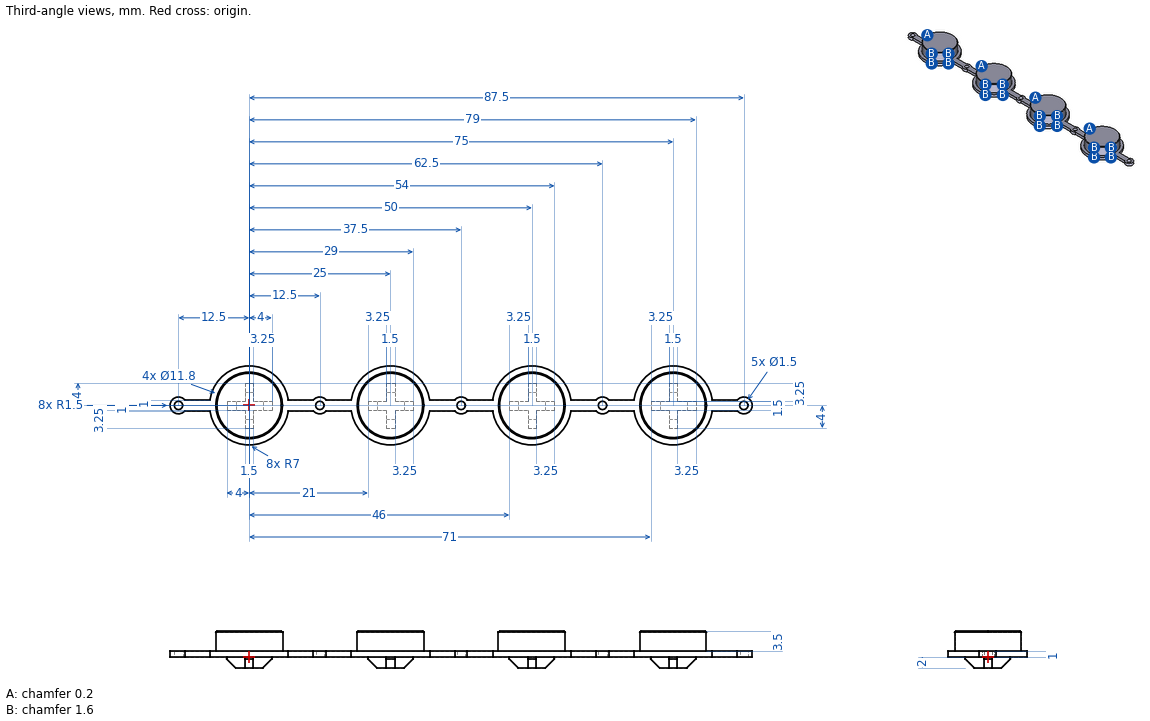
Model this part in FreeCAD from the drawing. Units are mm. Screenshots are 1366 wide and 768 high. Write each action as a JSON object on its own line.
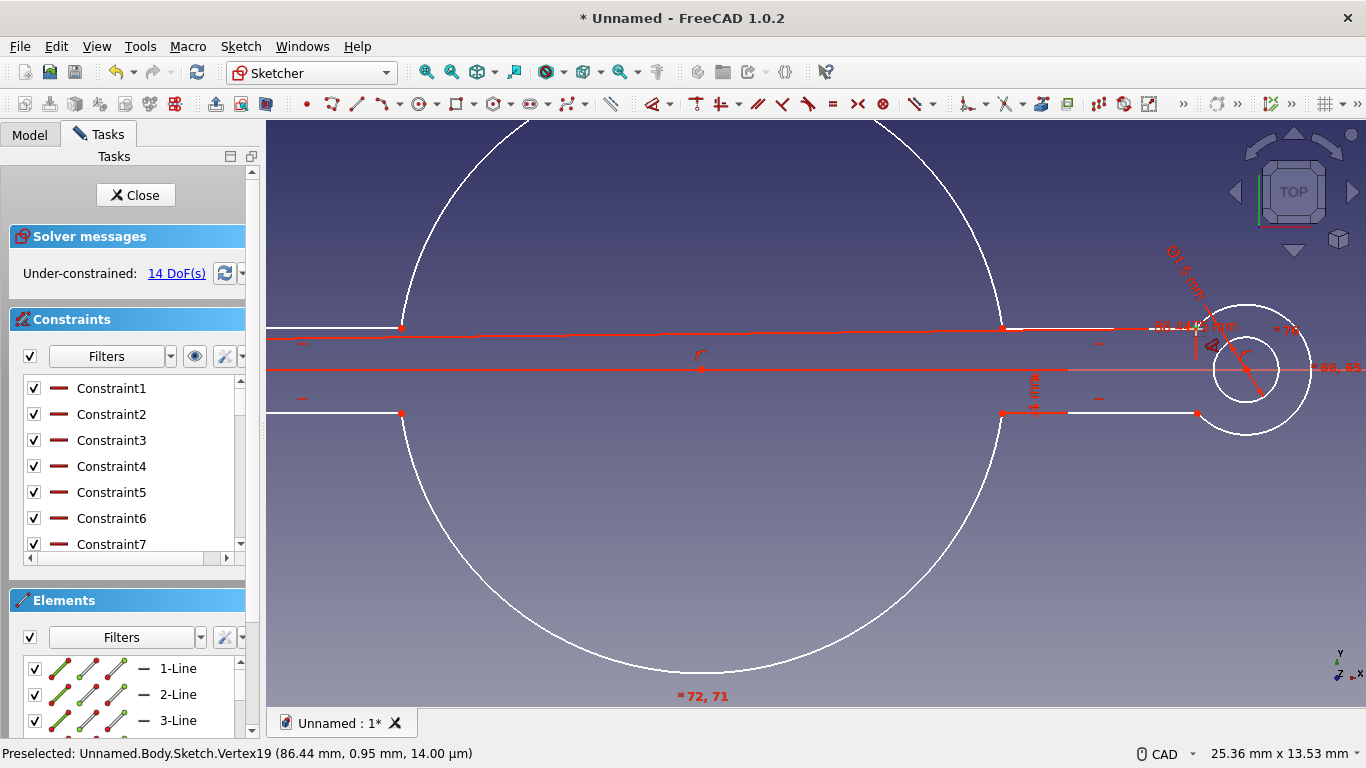
{"action": "key", "text": "Escape"}
{"action": "key", "text": "Escape"}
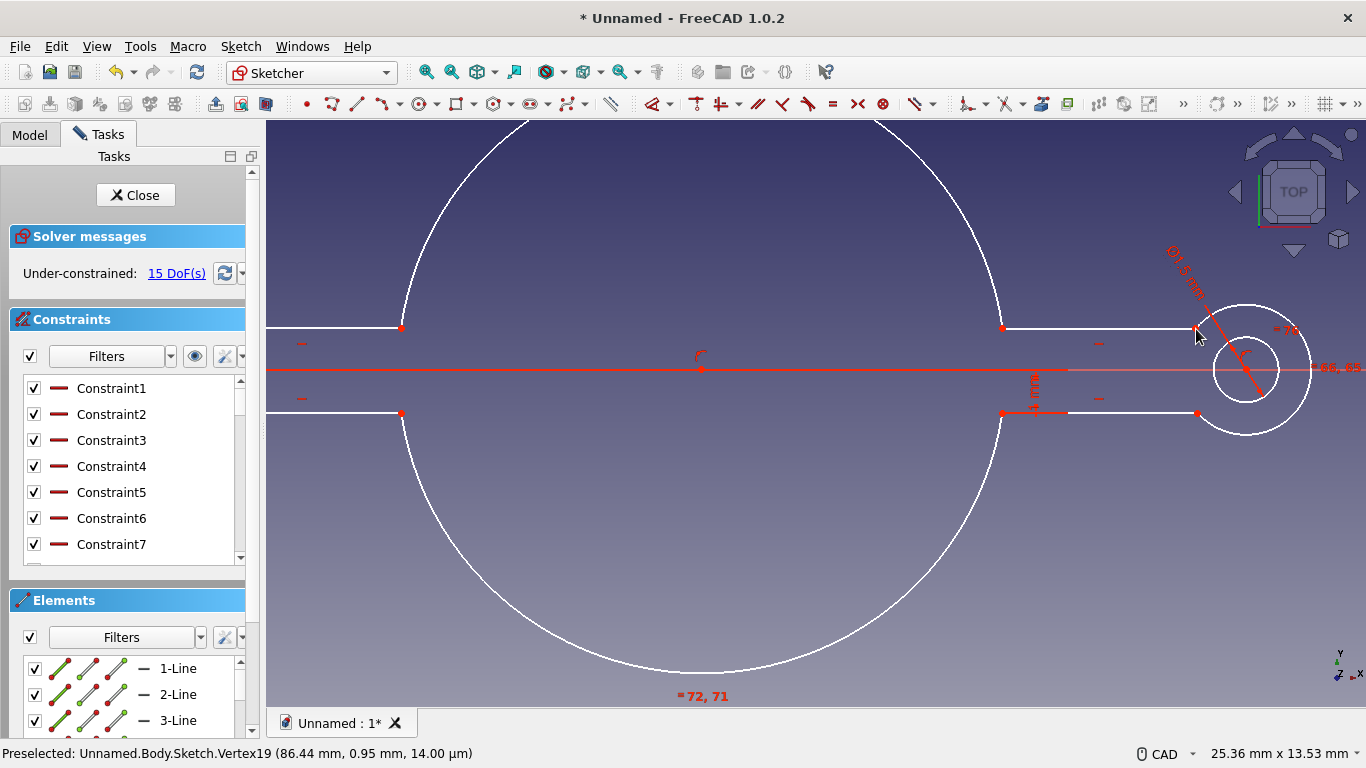
{"action": "left_click", "coordinate": [1196, 329]}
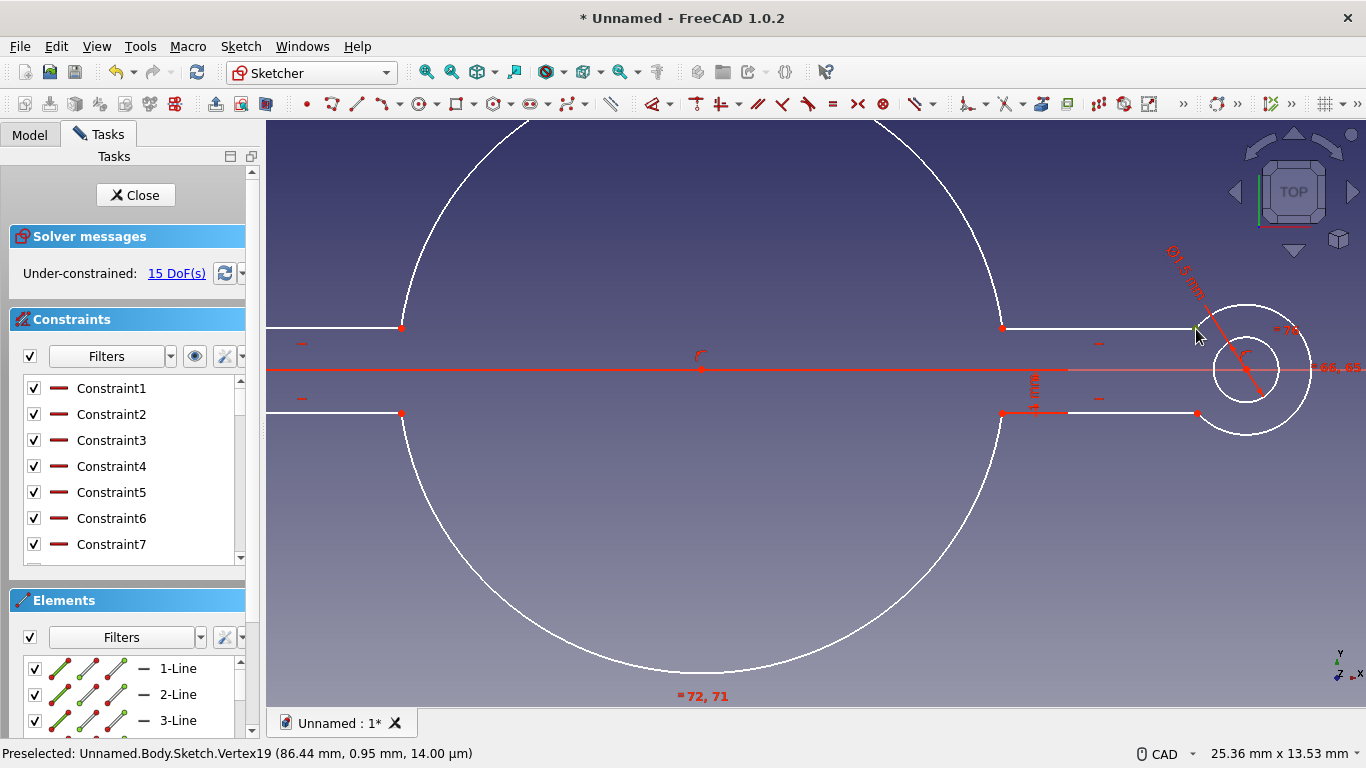
{"action": "key", "text": "i"}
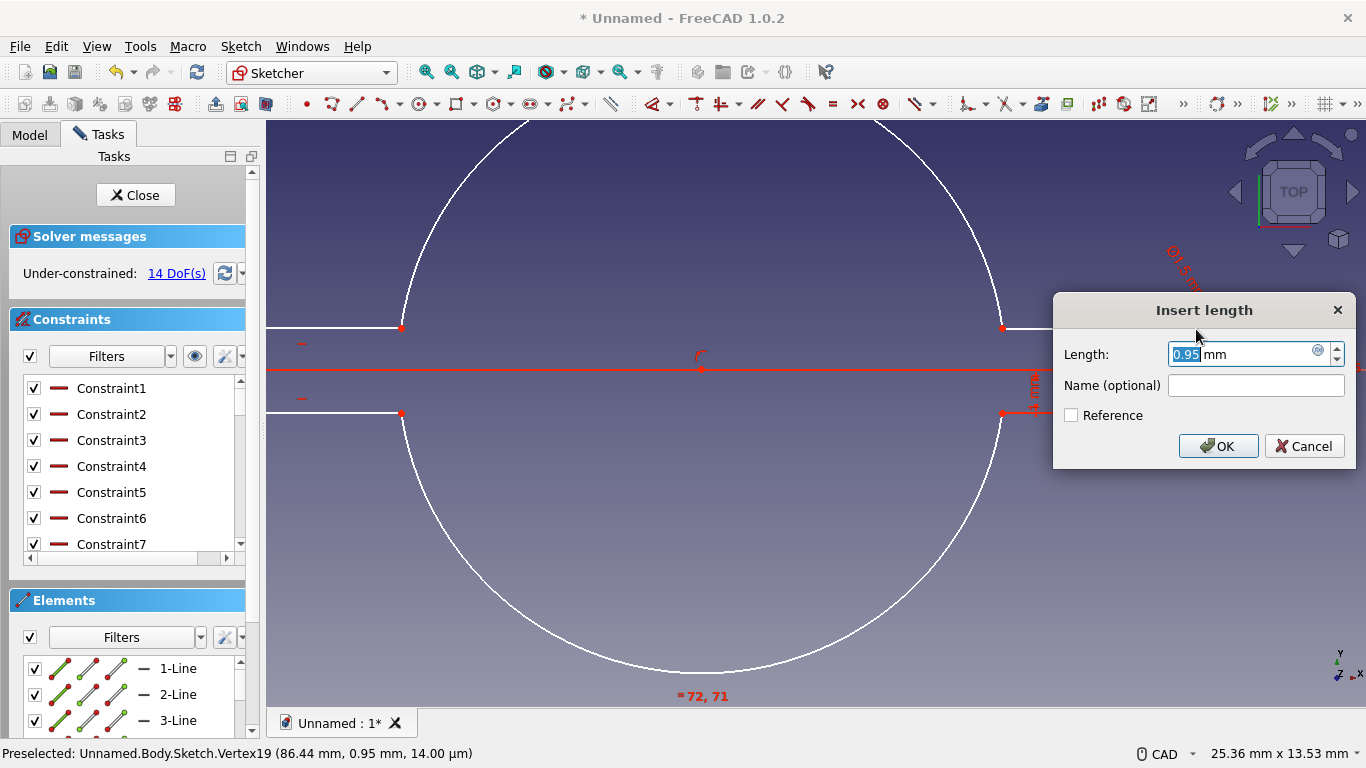
{"action": "type", "text": "1"}
{"action": "key", "text": "Return"}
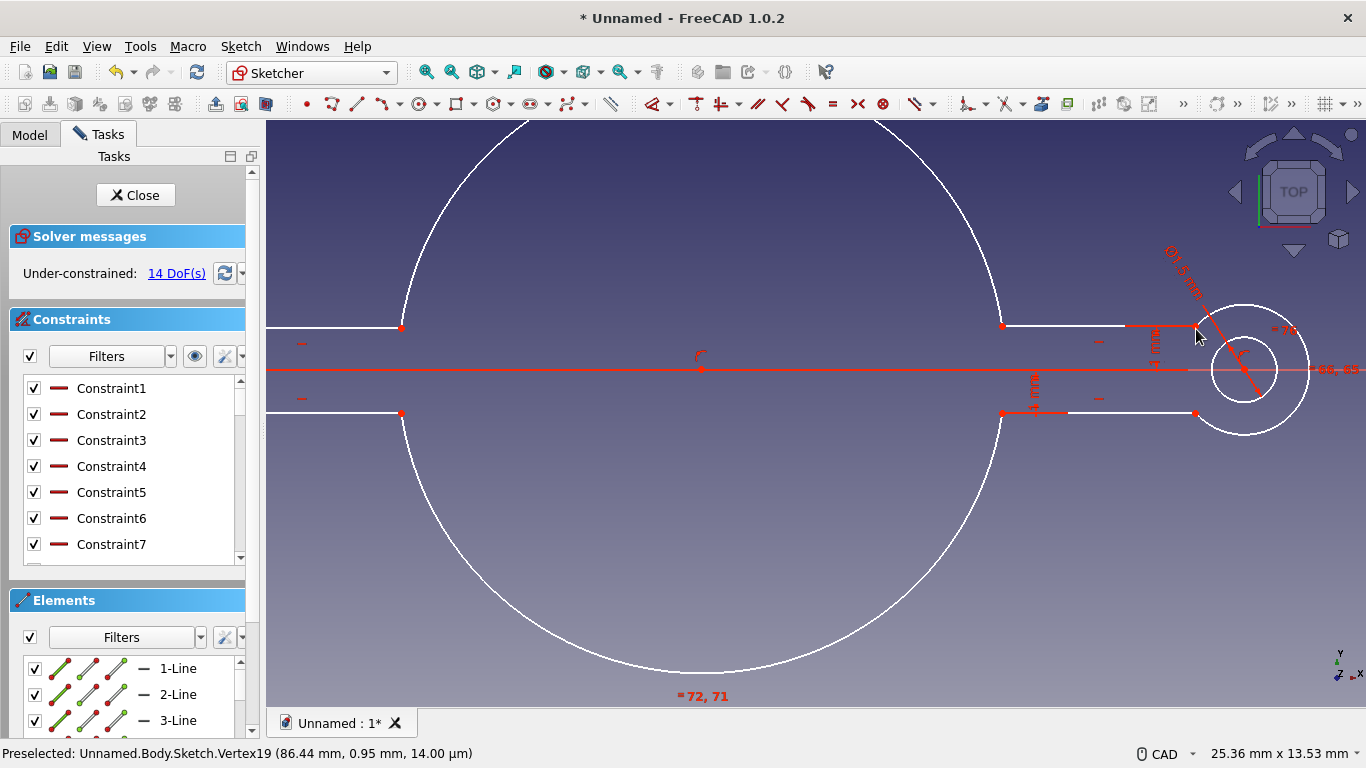
{"action": "left_click", "coordinate": [401, 328]}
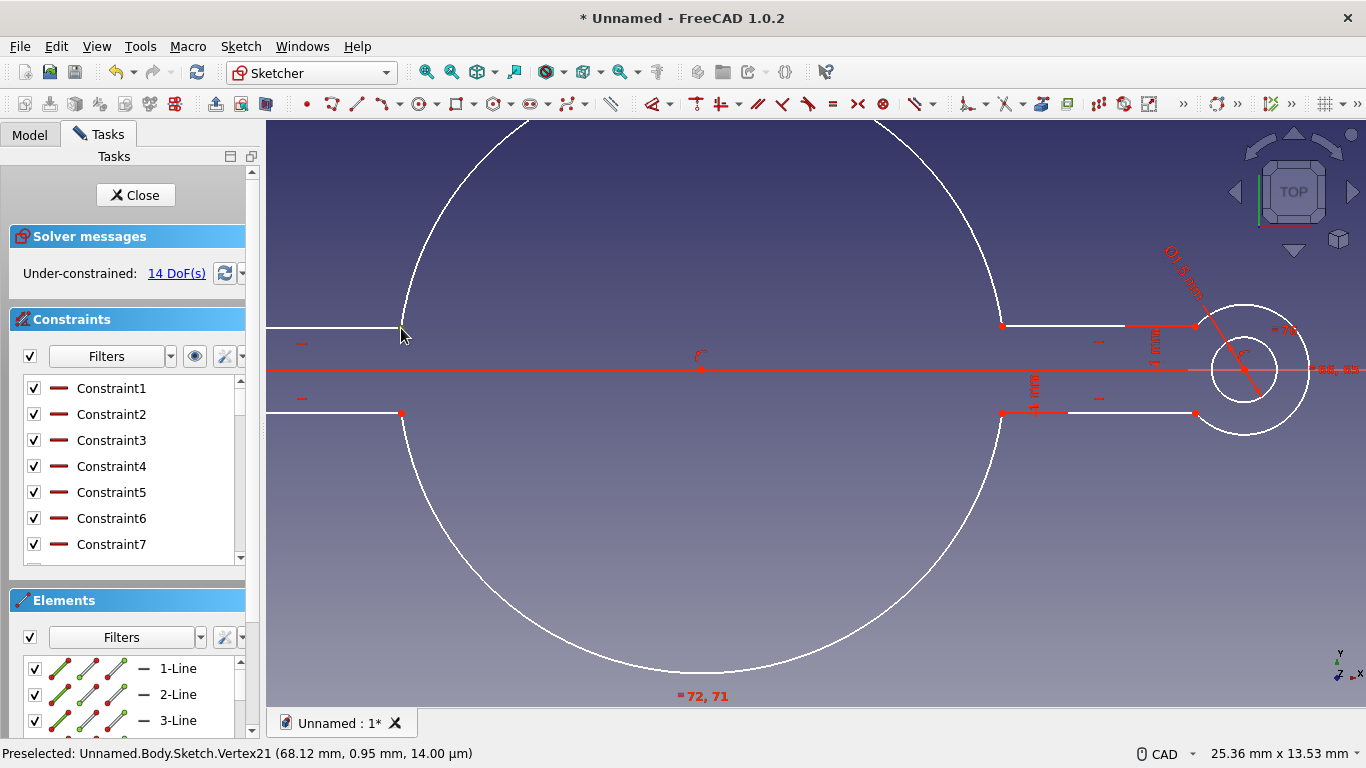
{"action": "left_click", "coordinate": [670, 104]}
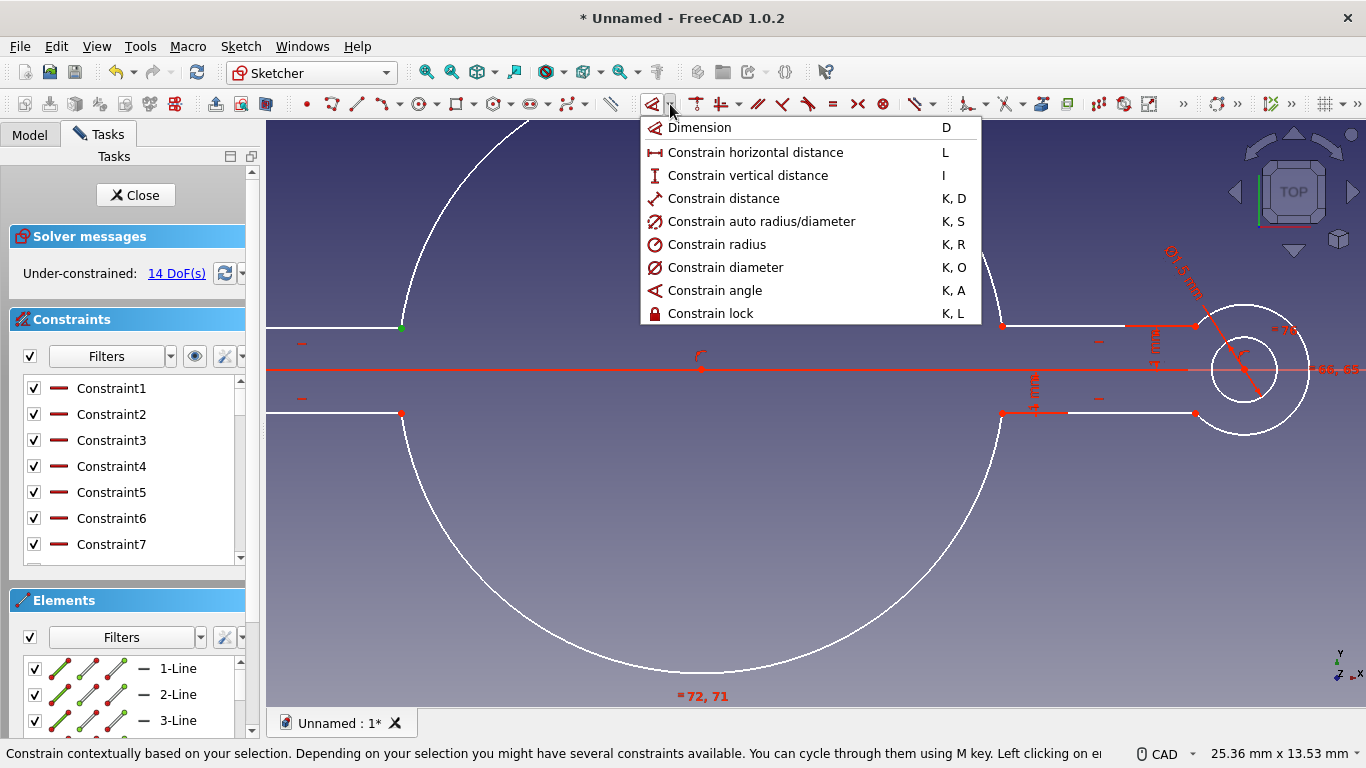
{"action": "left_click", "coordinate": [811, 176]}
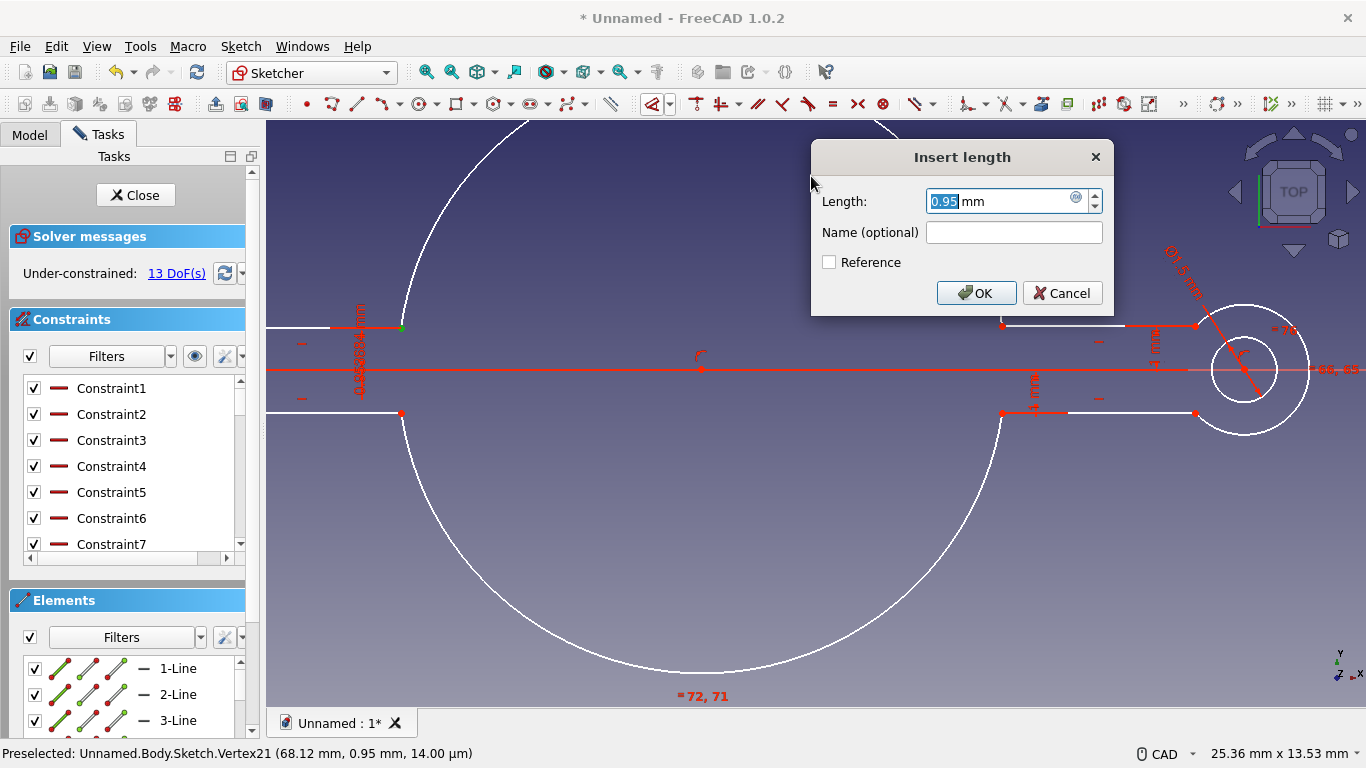
{"action": "type", "text": "1"}
{"action": "key", "text": "Return"}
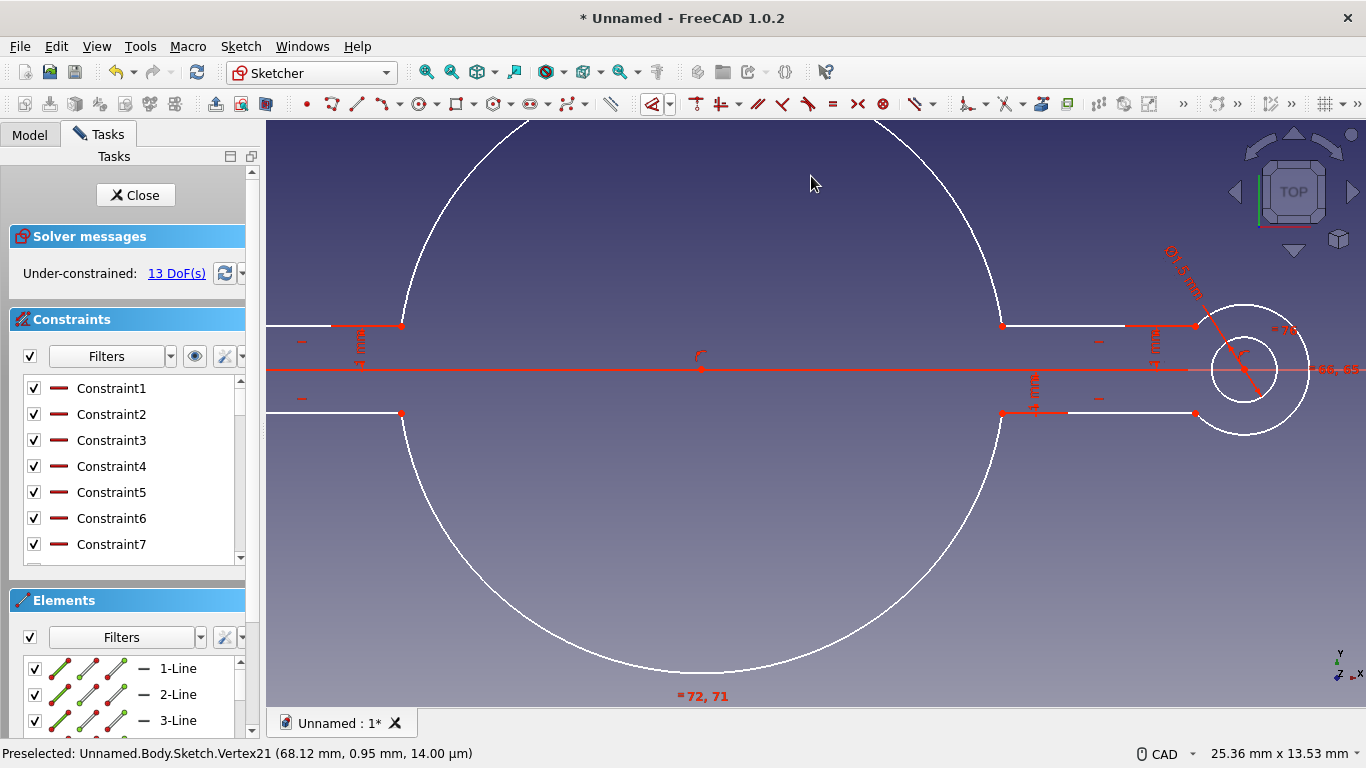
{"action": "scroll", "coordinate": [1010, 420], "scroll_direction": "down", "scroll_amount": 10}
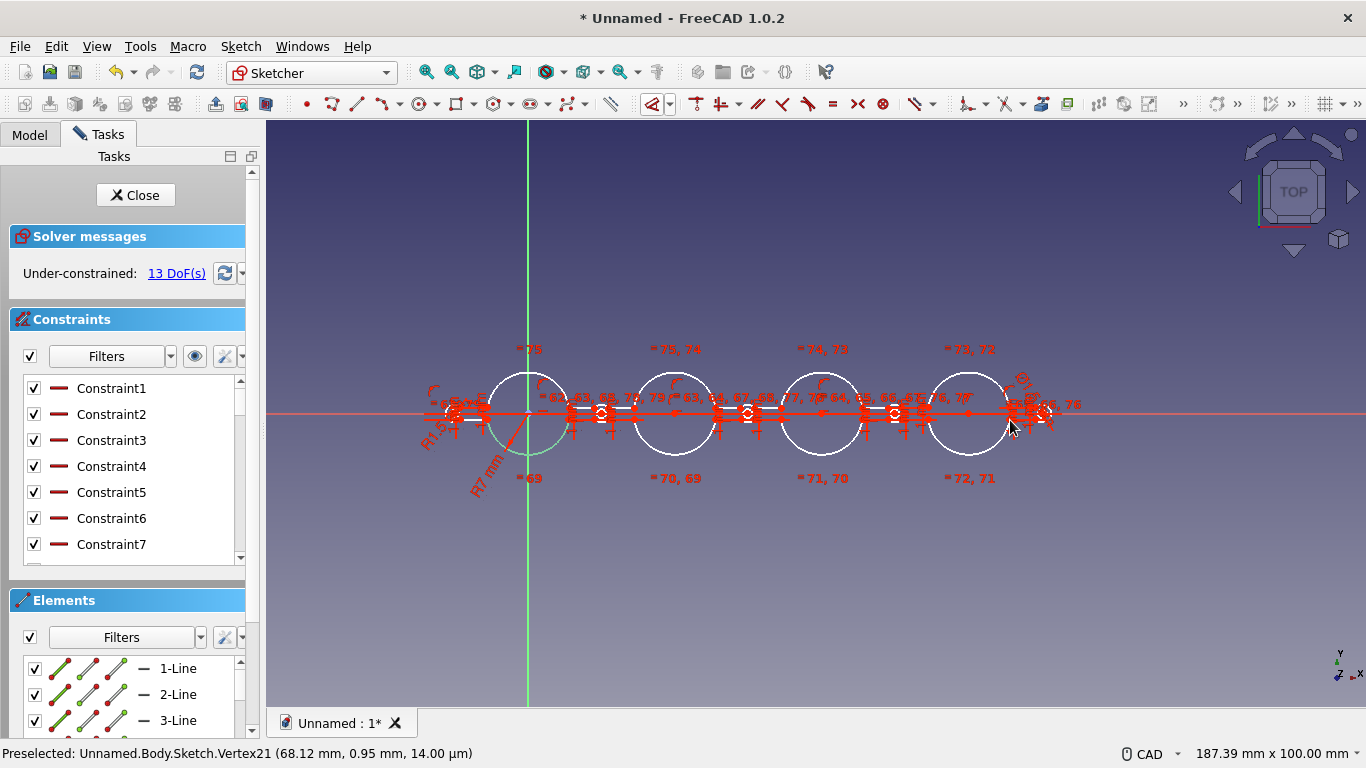
{"action": "scroll", "coordinate": [888, 408], "scroll_direction": "up", "scroll_amount": 10}